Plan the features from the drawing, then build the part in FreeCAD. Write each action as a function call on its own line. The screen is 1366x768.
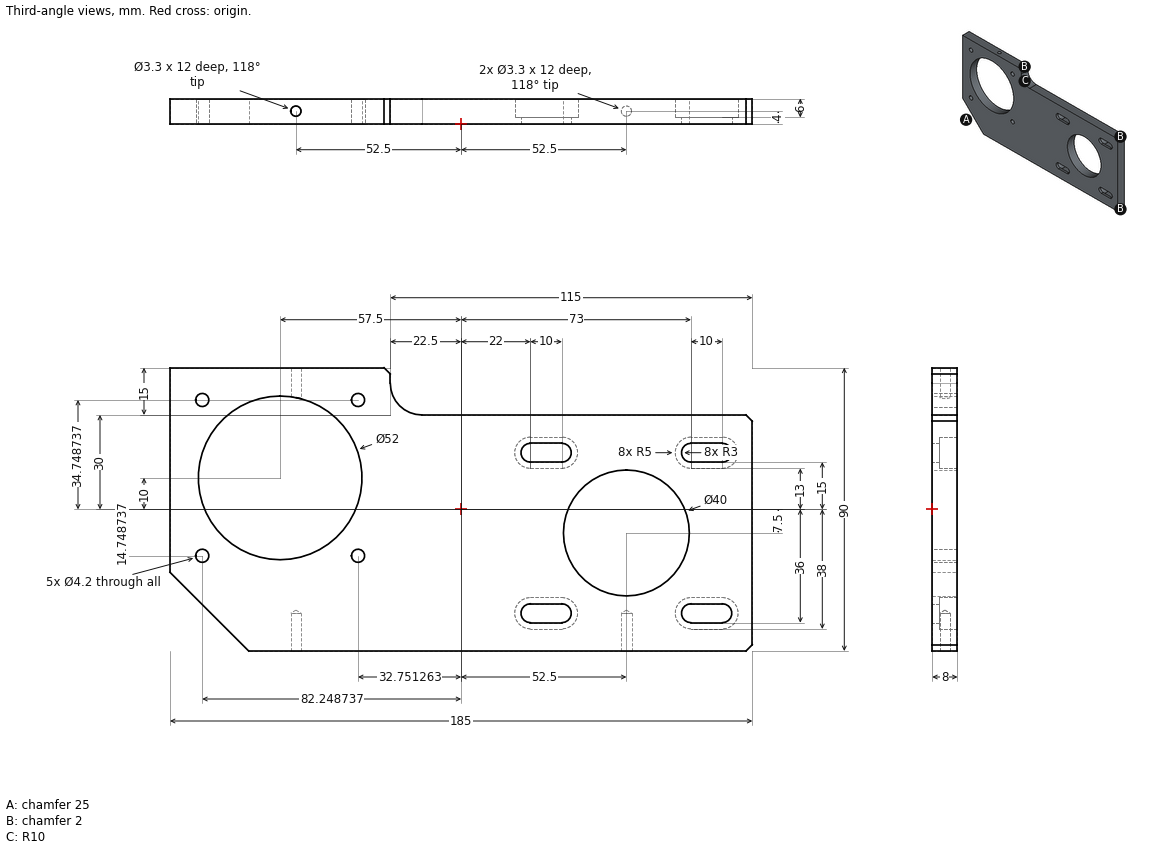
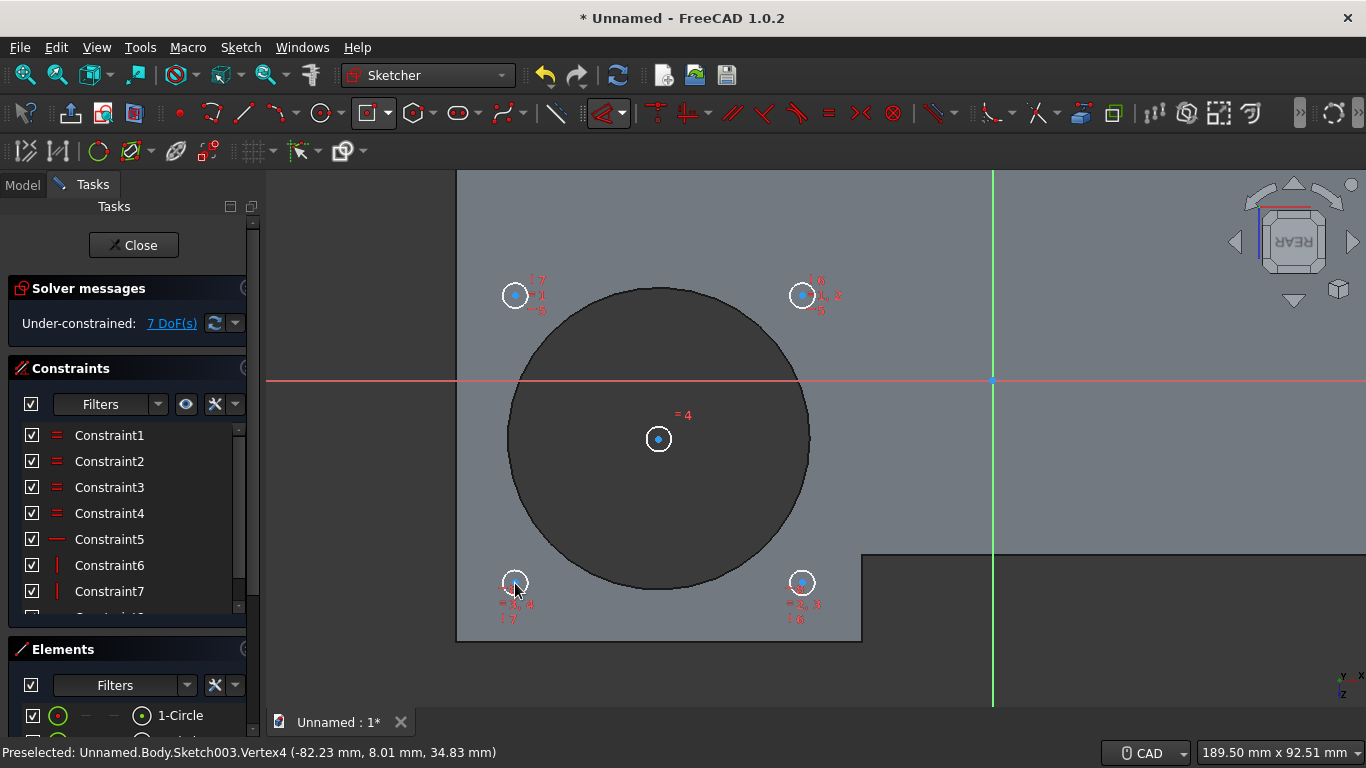
scroll(524, 287, up, 3)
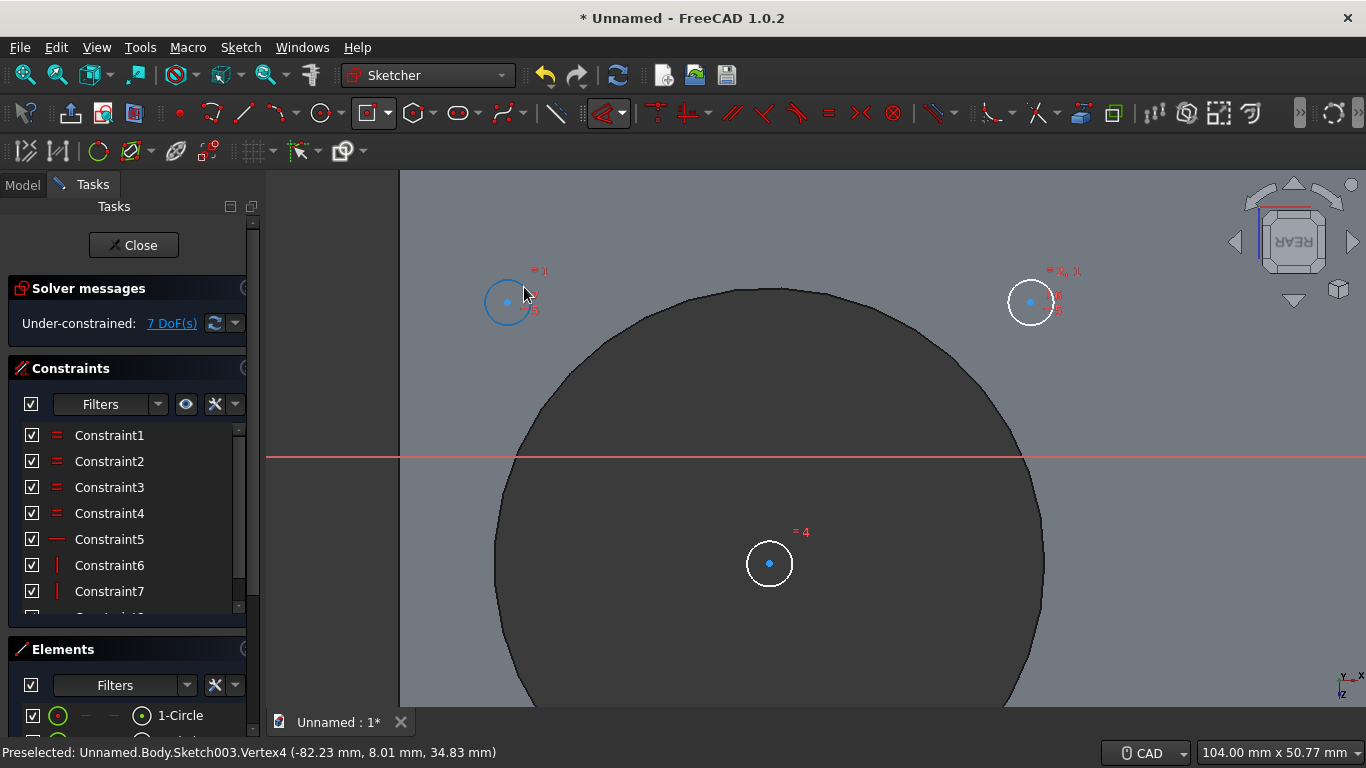
click(492, 287)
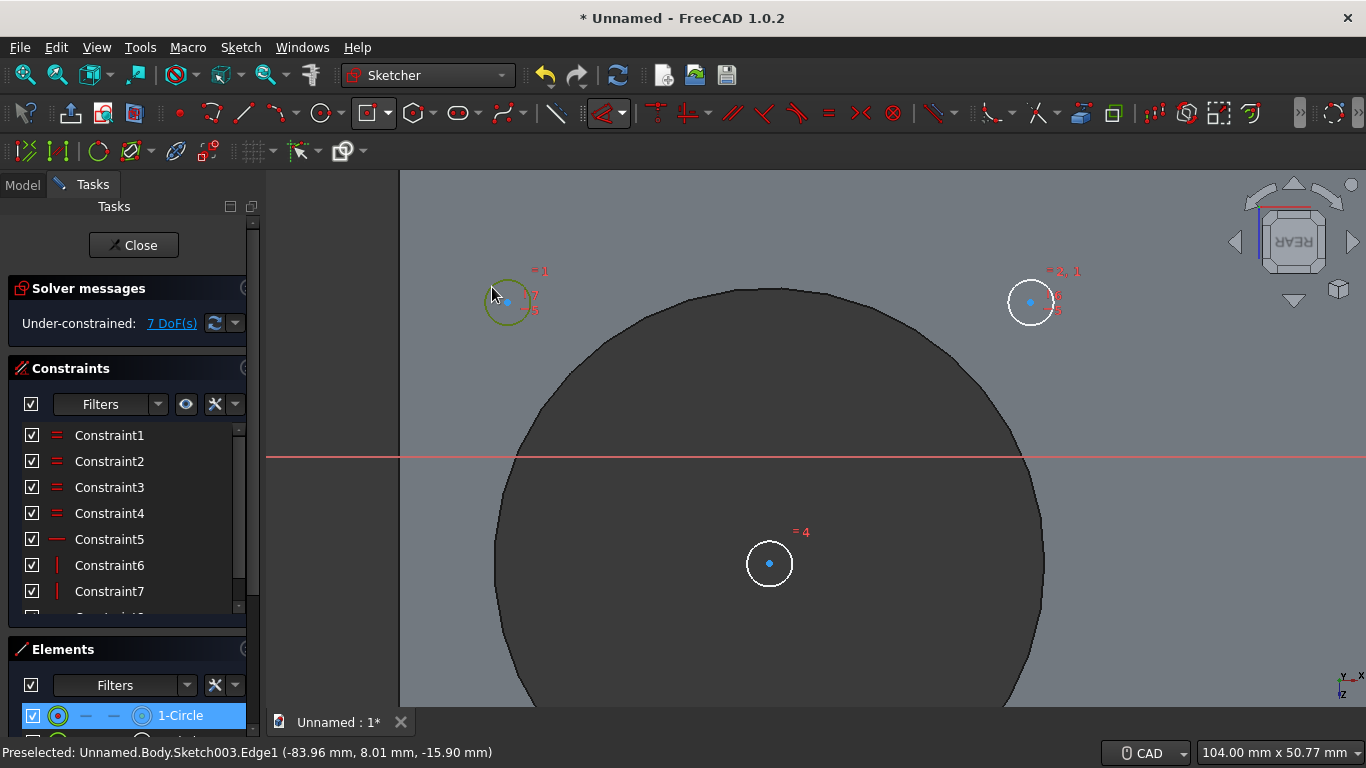
key(k)
key(o)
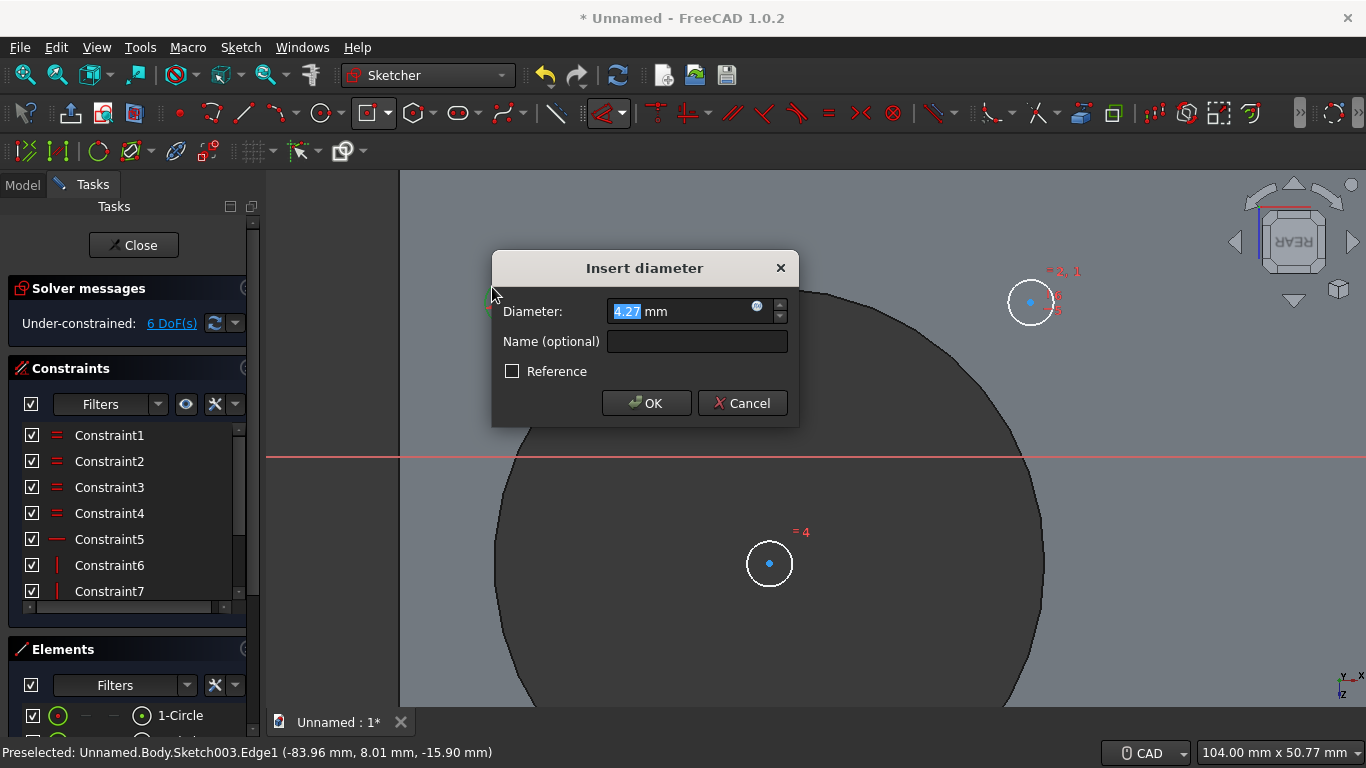
text(4.2)
key(Return)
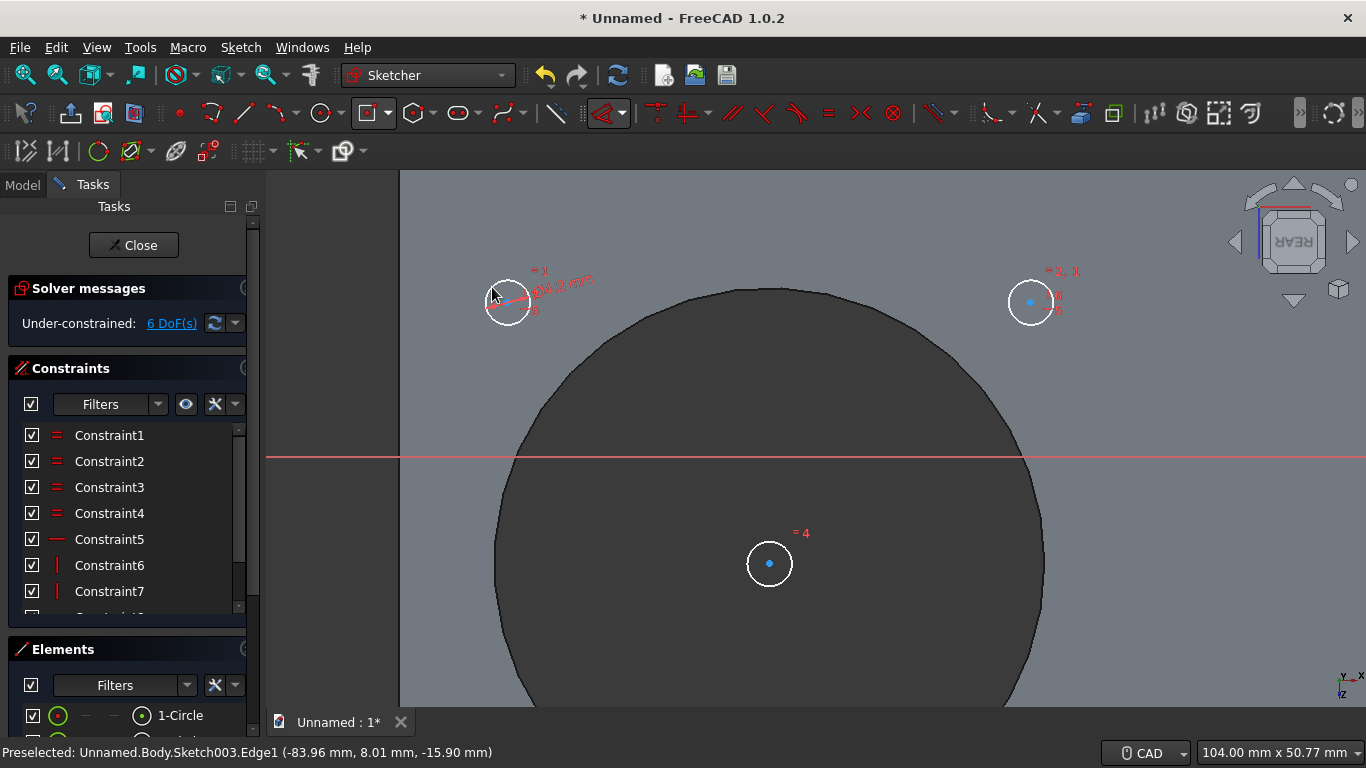
click(770, 564)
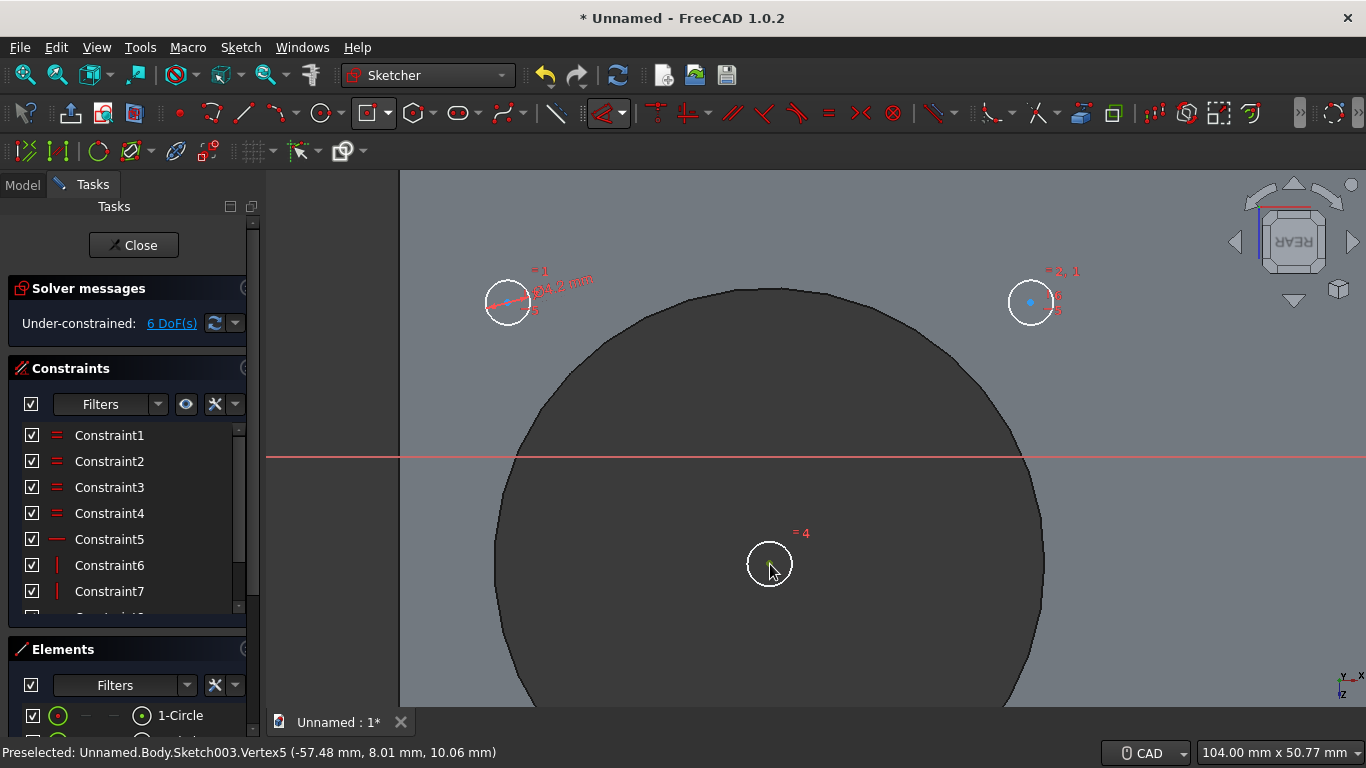
key(i)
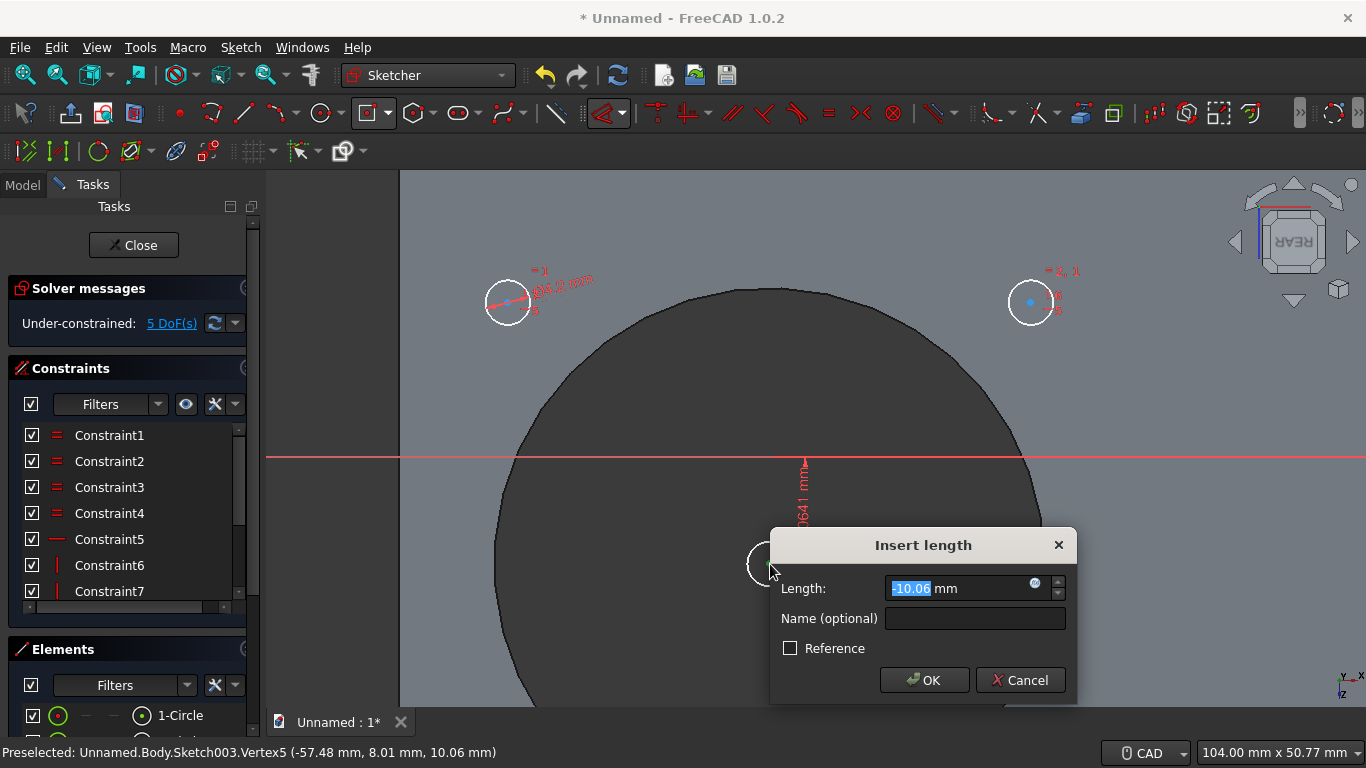
text(-10)
key(Return)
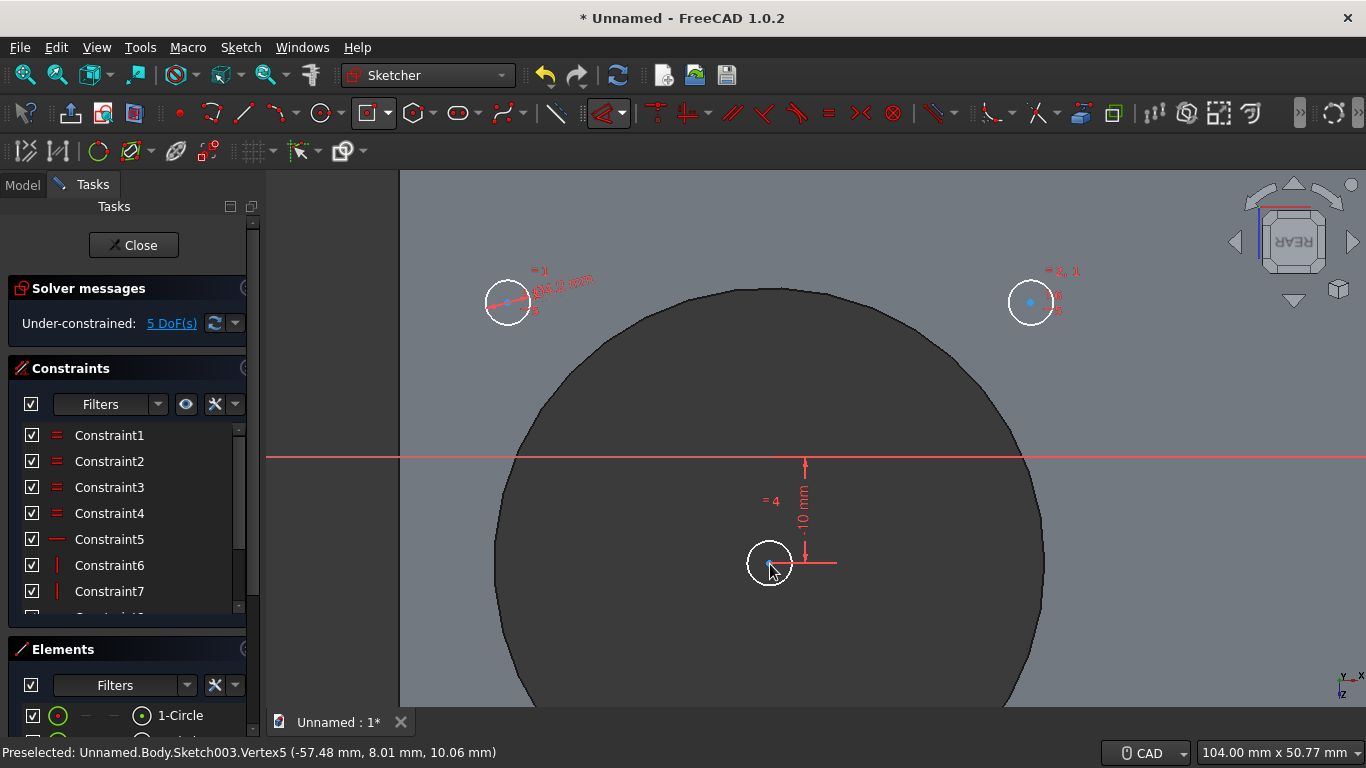
click(770, 563)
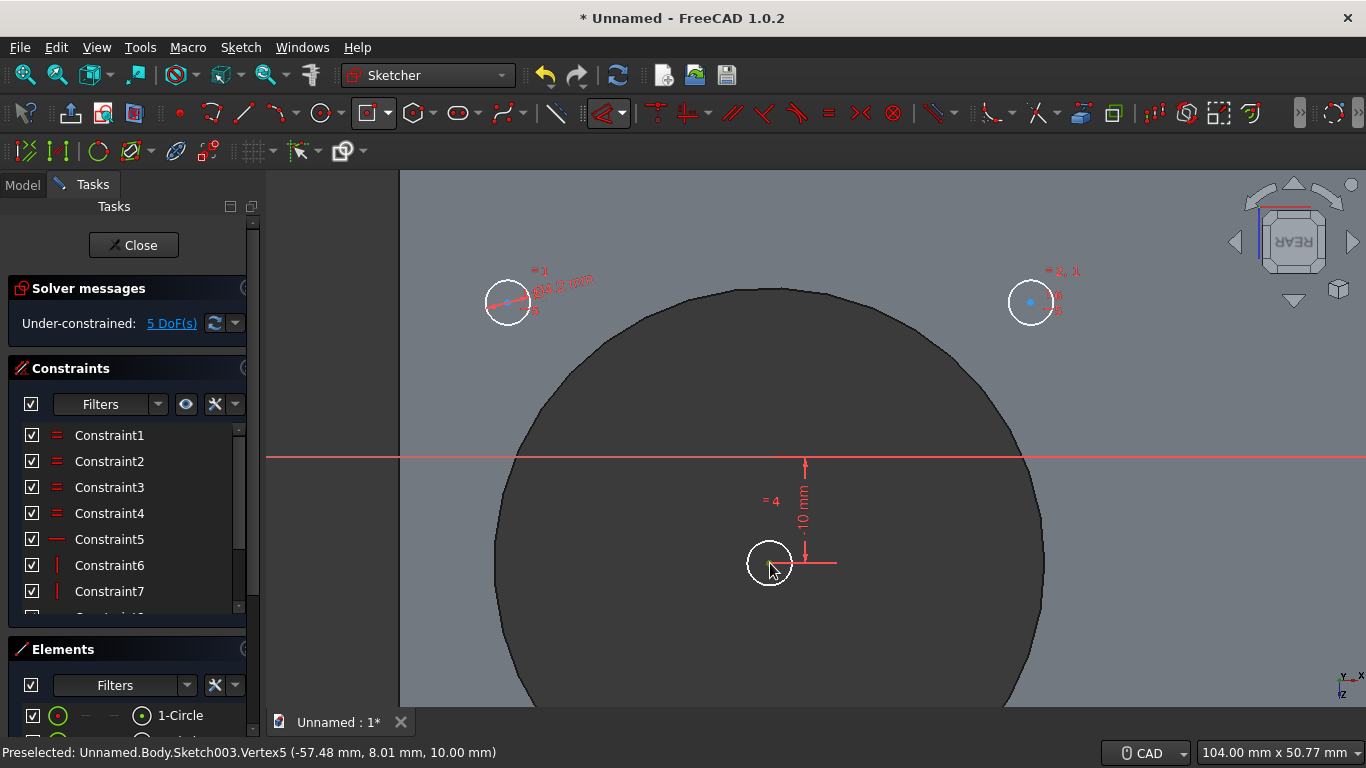
click(624, 114)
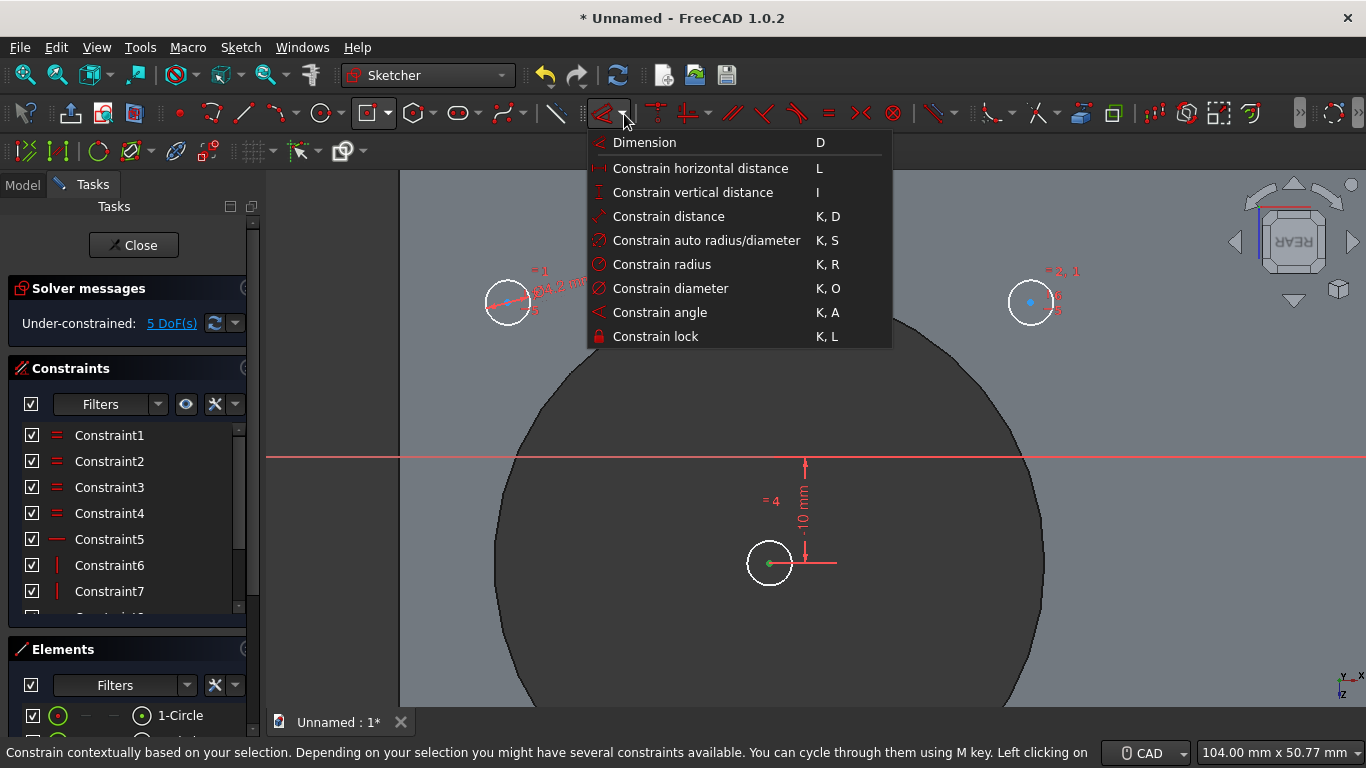
click(740, 168)